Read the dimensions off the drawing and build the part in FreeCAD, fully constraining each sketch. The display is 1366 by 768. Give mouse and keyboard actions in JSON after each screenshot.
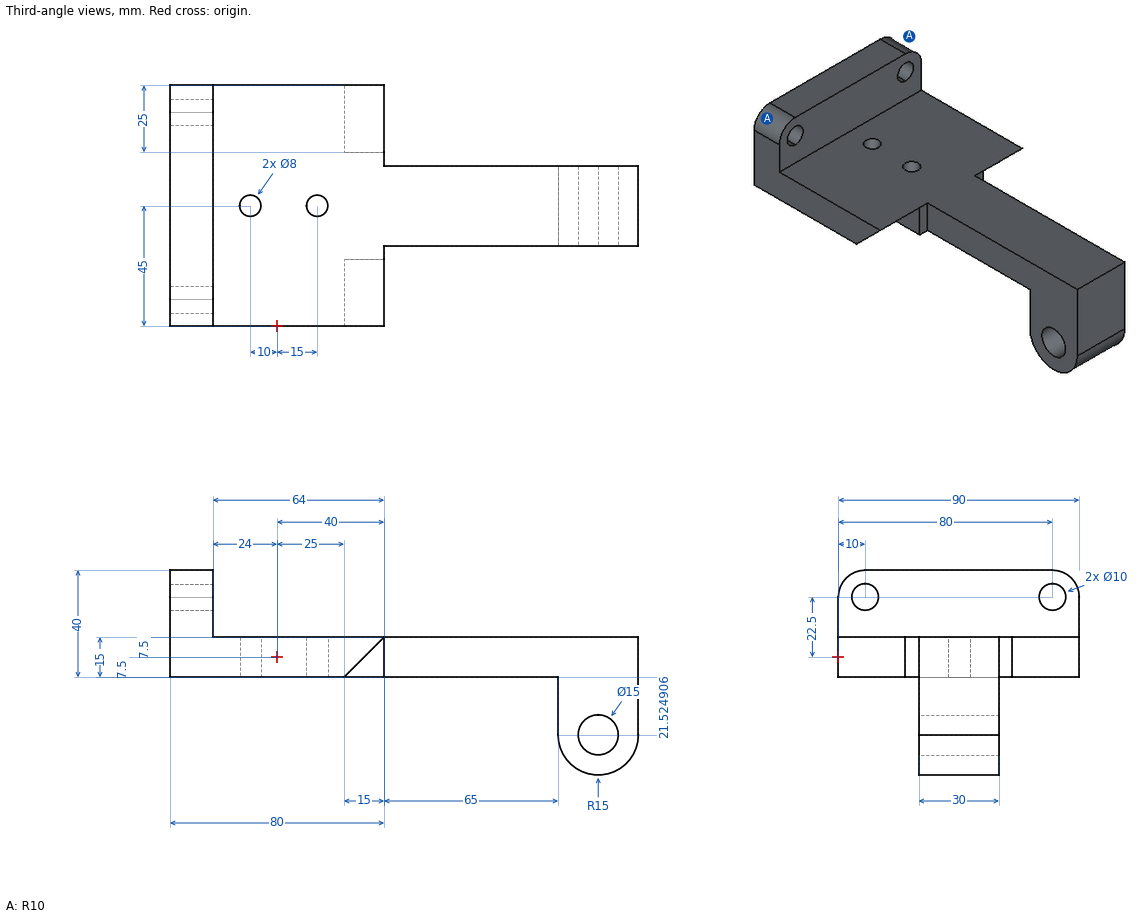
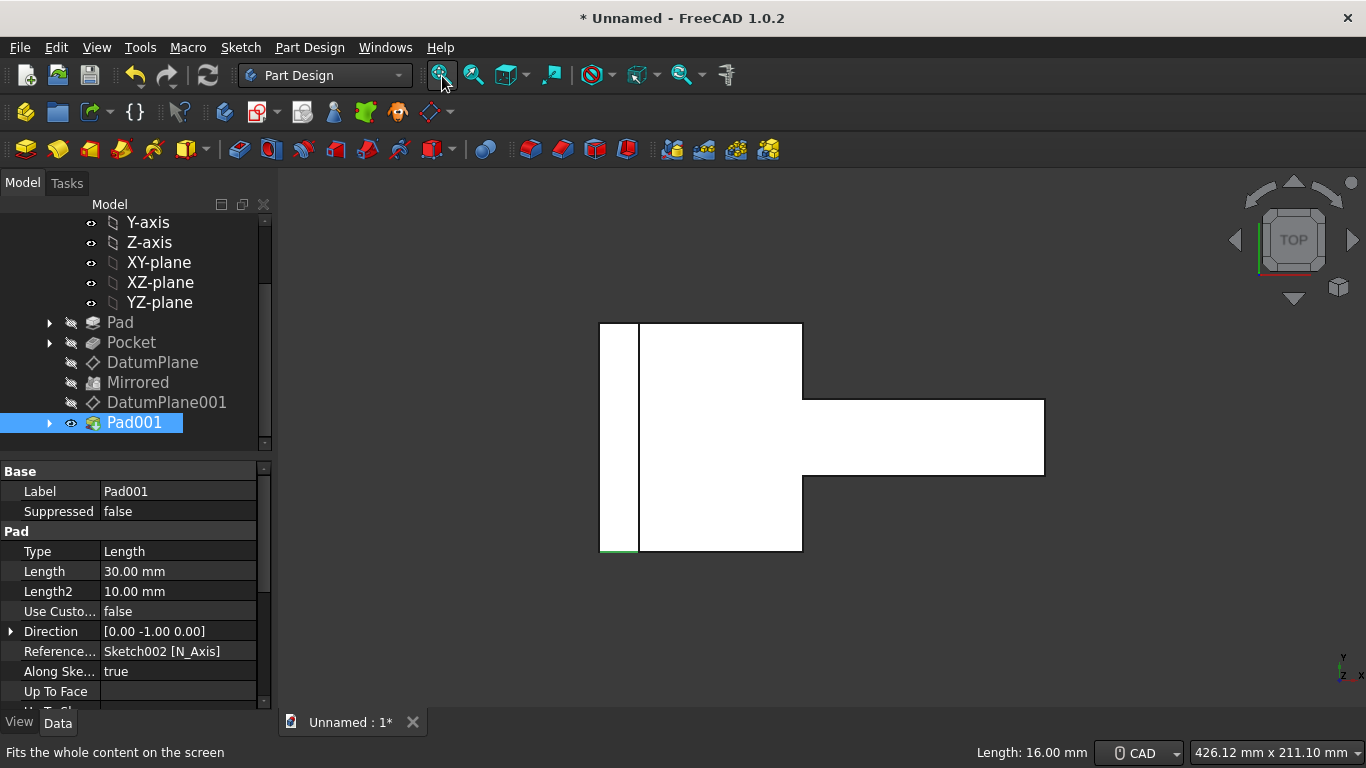
{"action": "left_click", "coordinate": [619, 322], "text": "ctrl"}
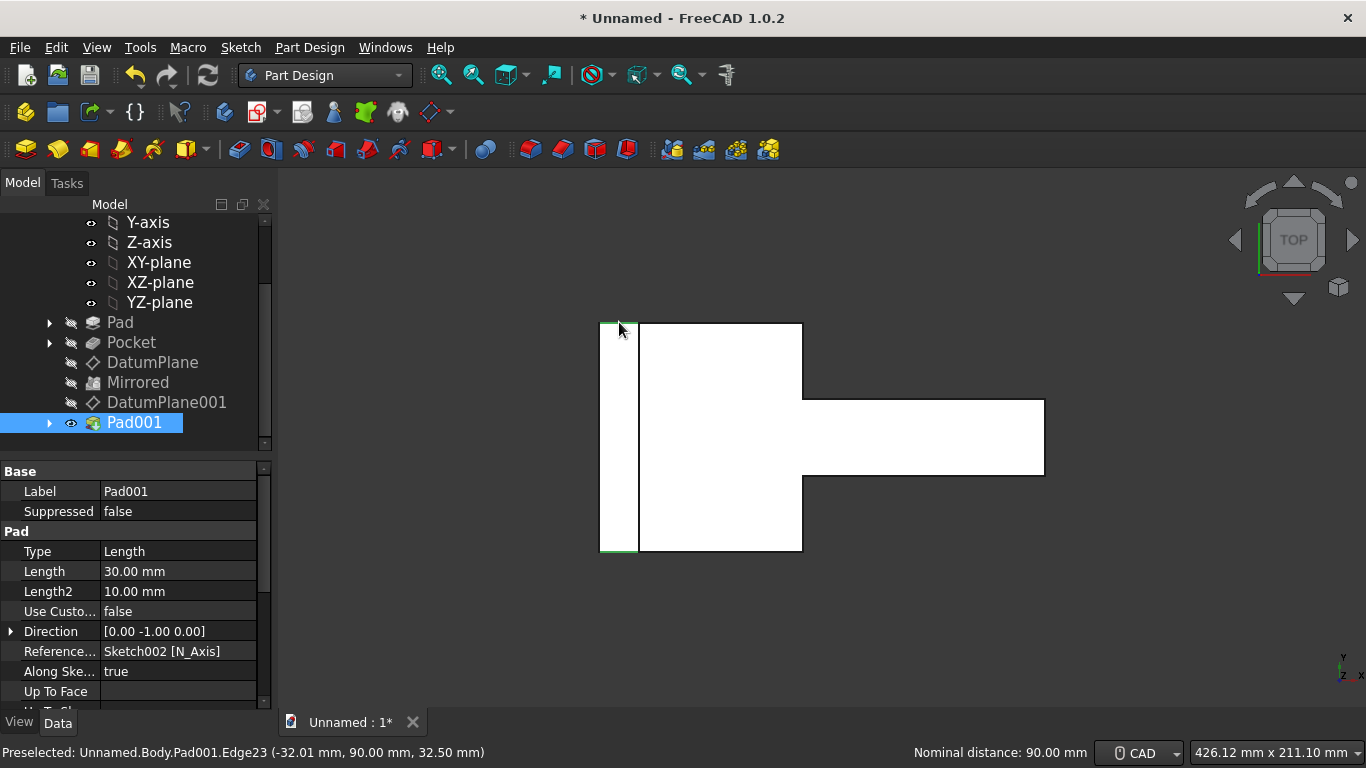
{"action": "left_click", "coordinate": [532, 150]}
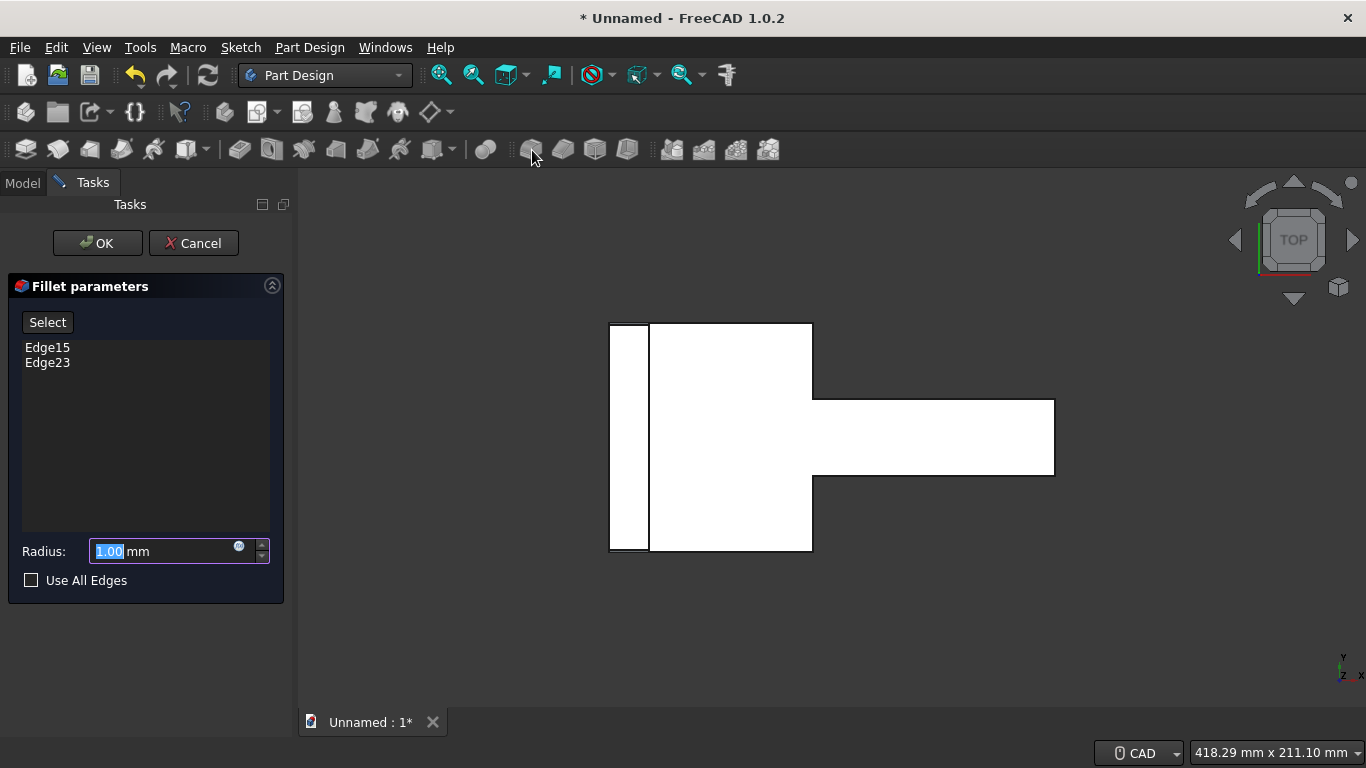
{"action": "type", "text": "10"}
{"action": "key", "text": "Tab"}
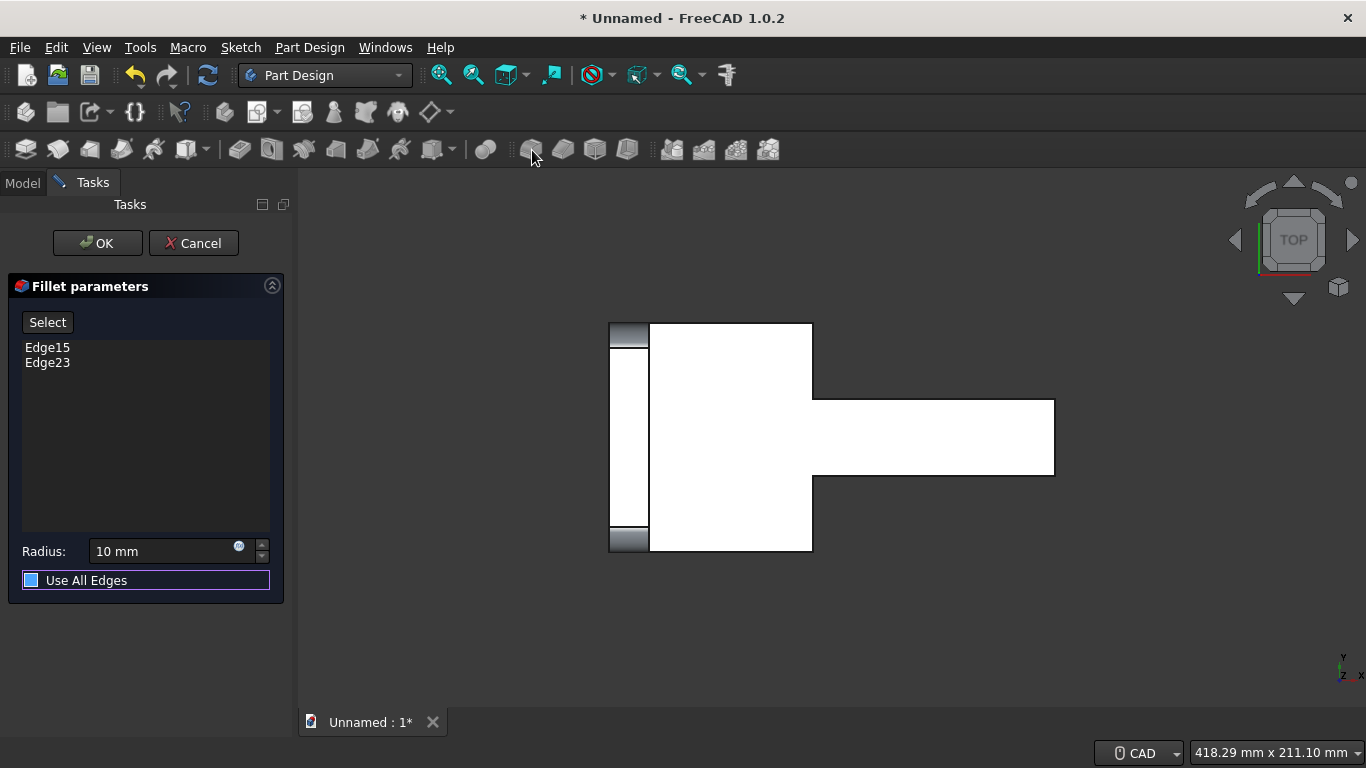
{"action": "left_click", "coordinate": [98, 243]}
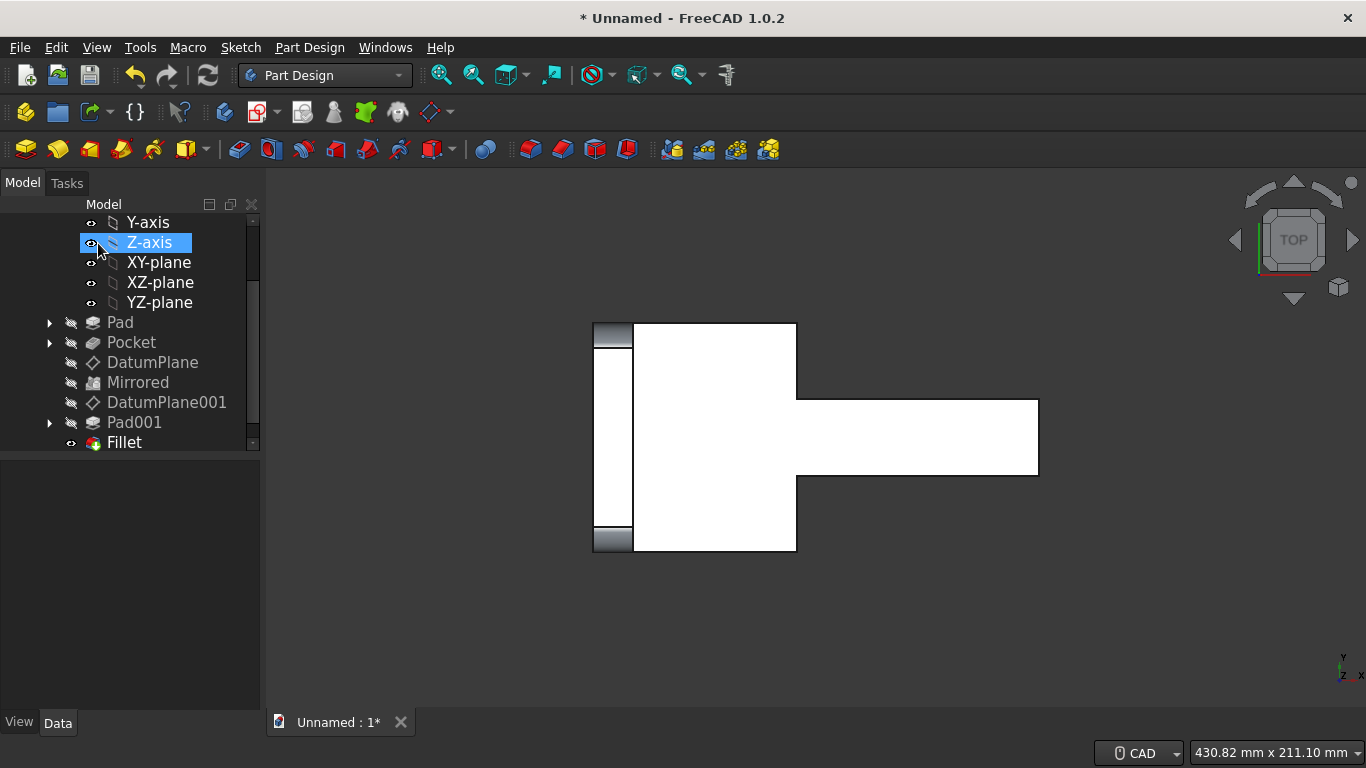
{"action": "left_click", "coordinate": [442, 76]}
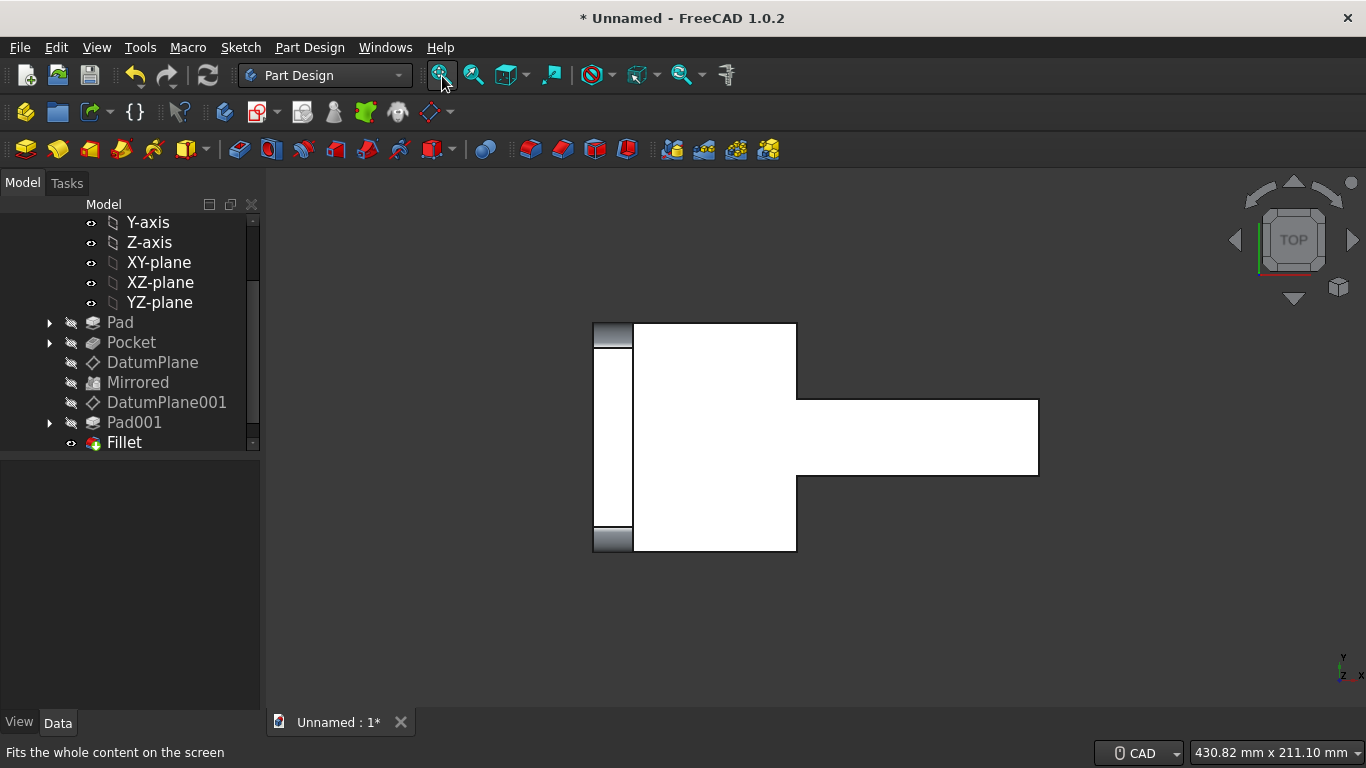
{"action": "key", "text": "6"}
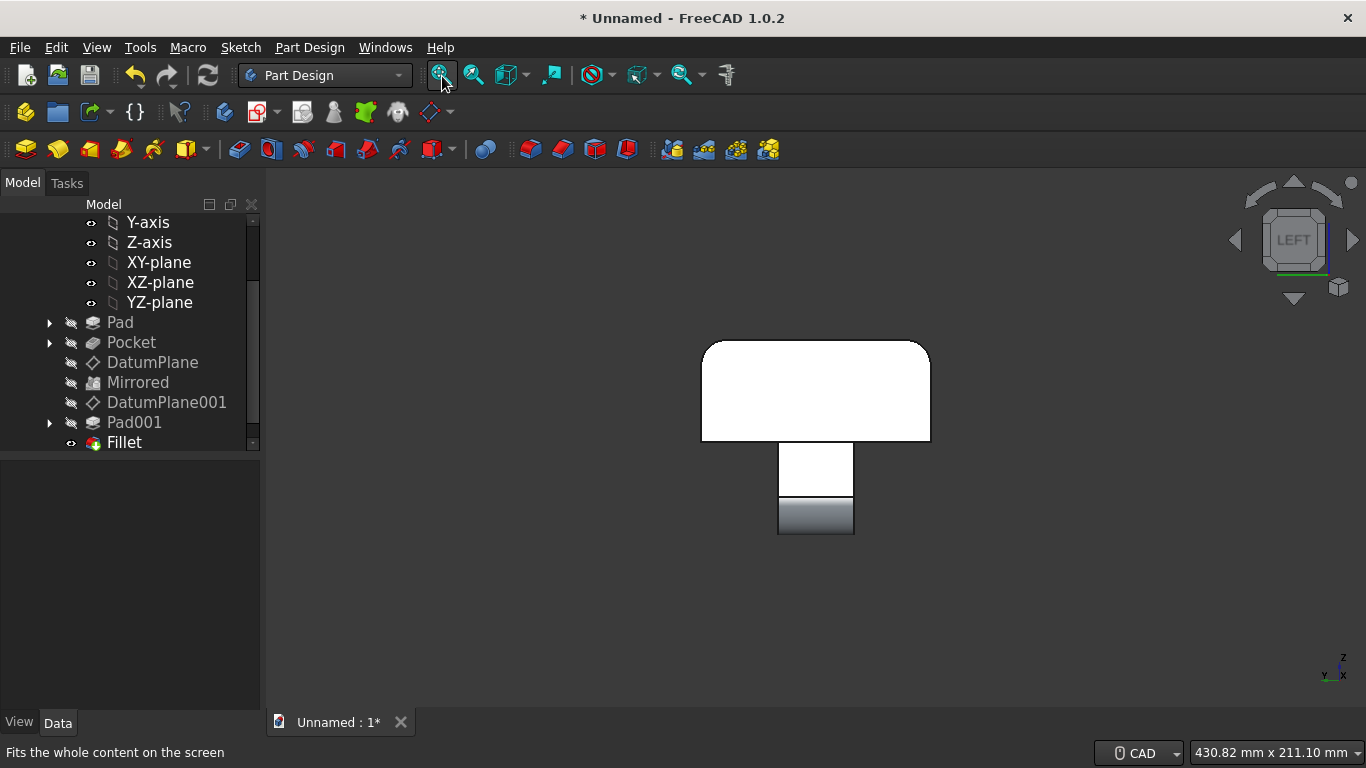
{"action": "left_click", "coordinate": [442, 76]}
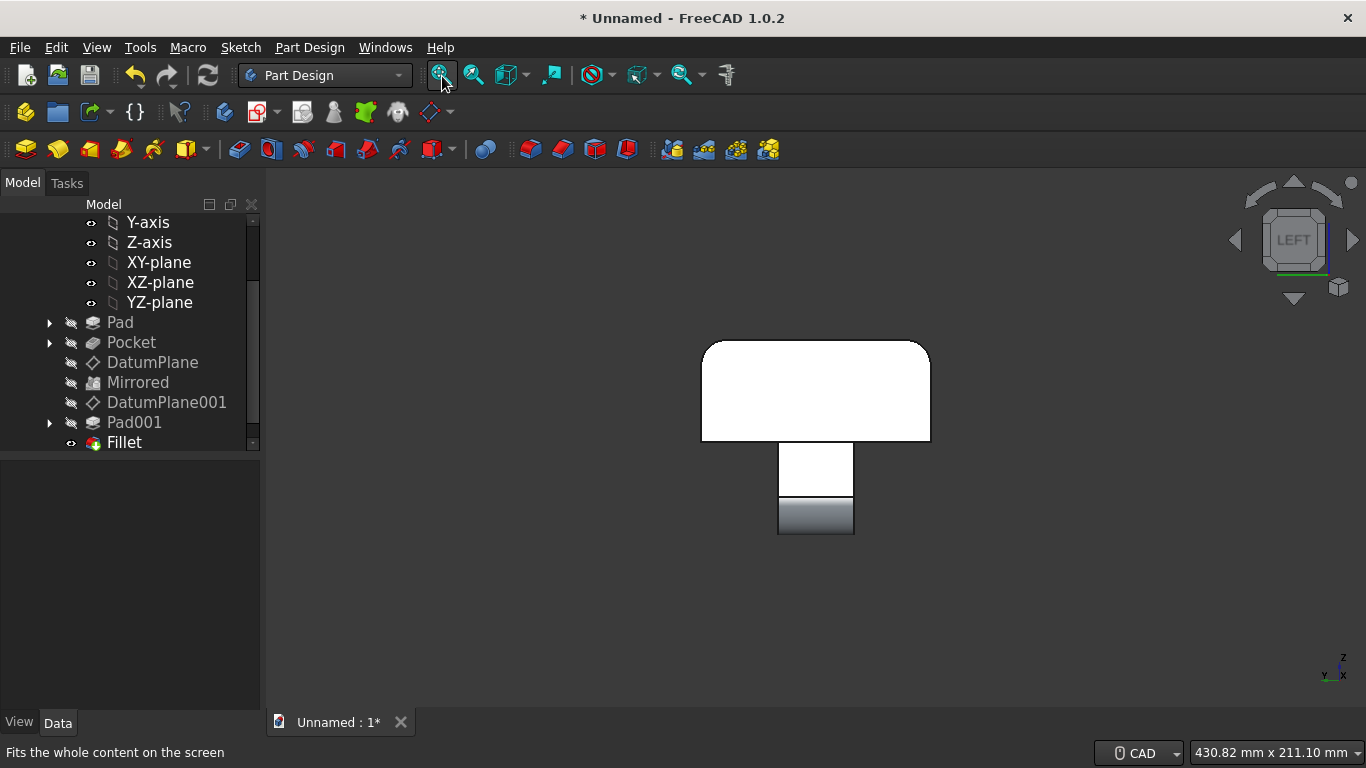
{"action": "left_click", "coordinate": [816, 390]}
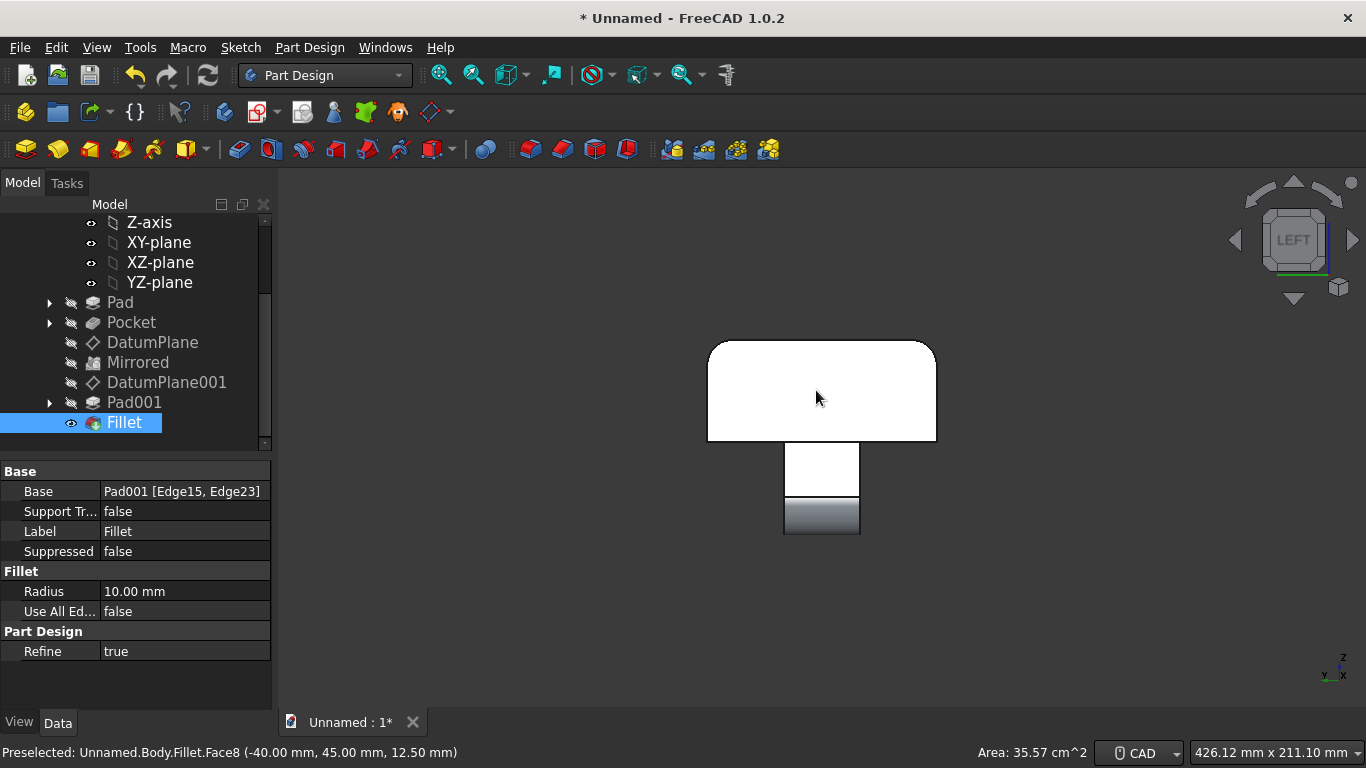
{"action": "left_click", "coordinate": [258, 112]}